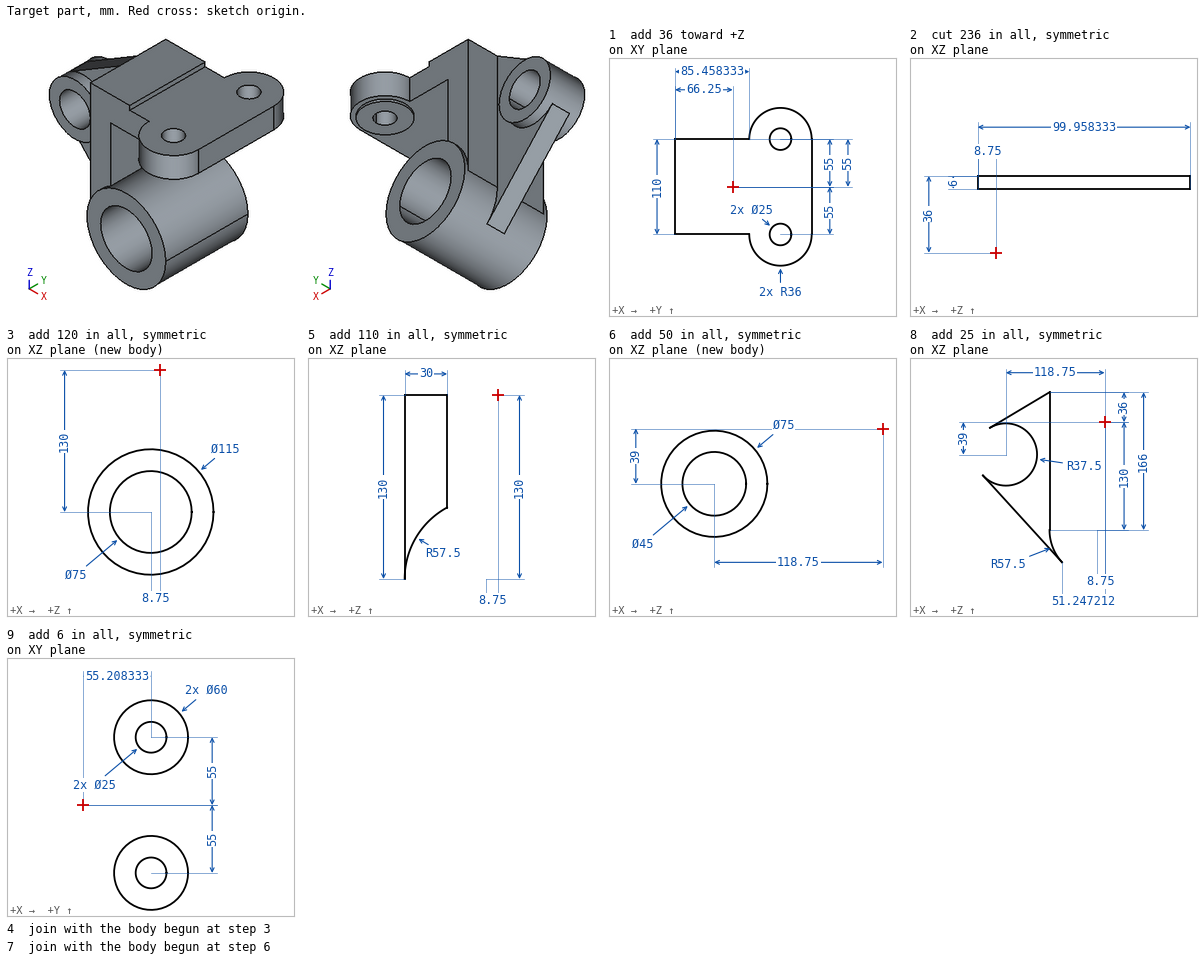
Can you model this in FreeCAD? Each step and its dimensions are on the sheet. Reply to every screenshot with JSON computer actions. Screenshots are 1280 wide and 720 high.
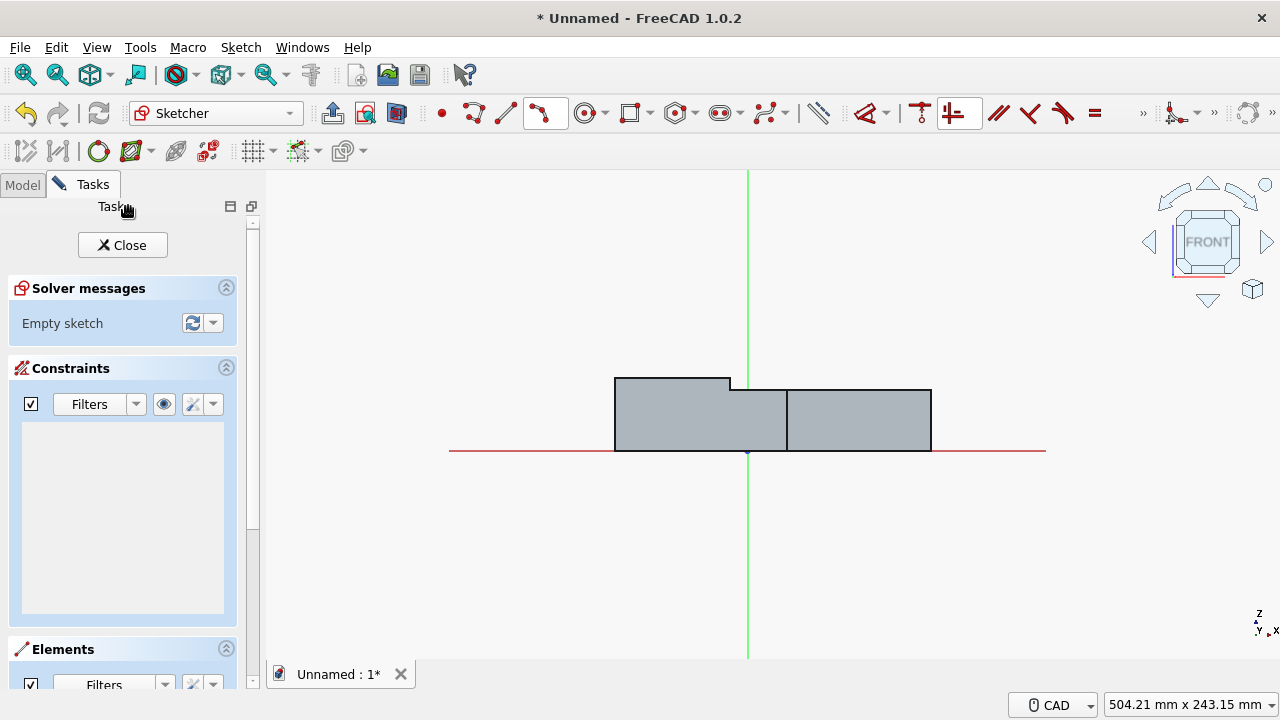
{"action": "scroll", "coordinate": [673, 198], "scroll_direction": "down", "scroll_amount": 3}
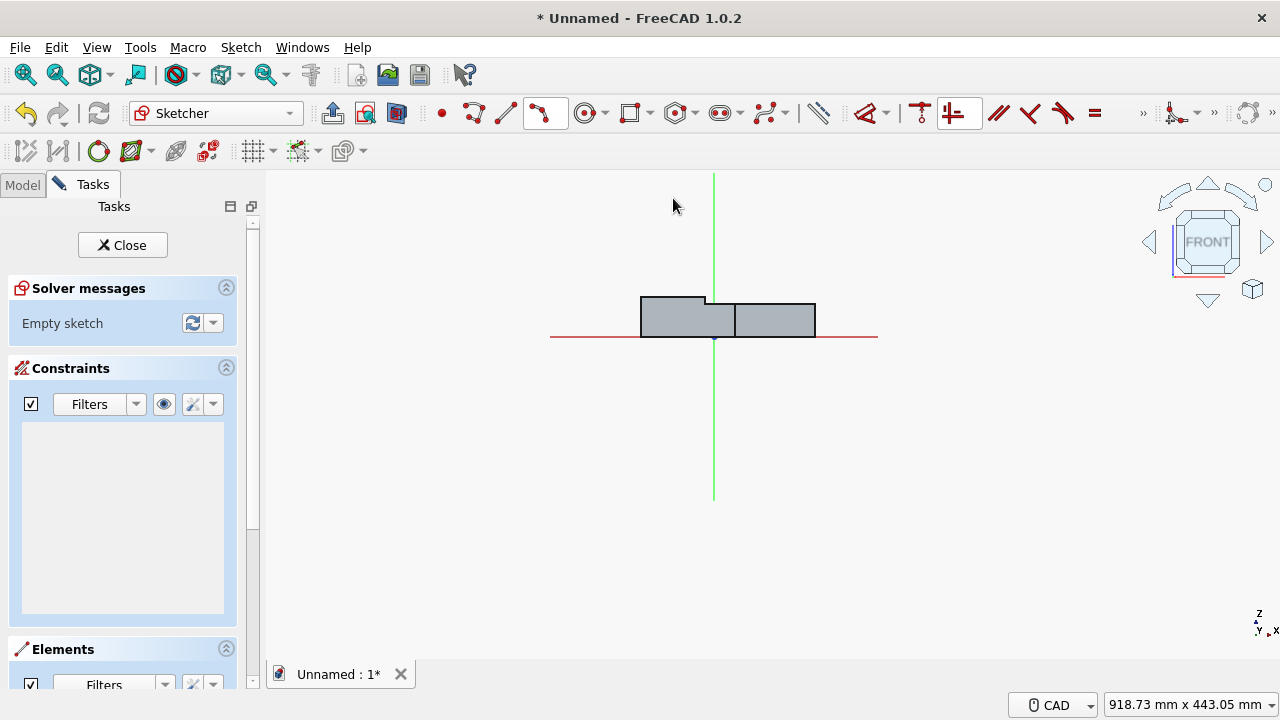
{"action": "scroll", "coordinate": [705, 492], "scroll_direction": "up", "scroll_amount": 2}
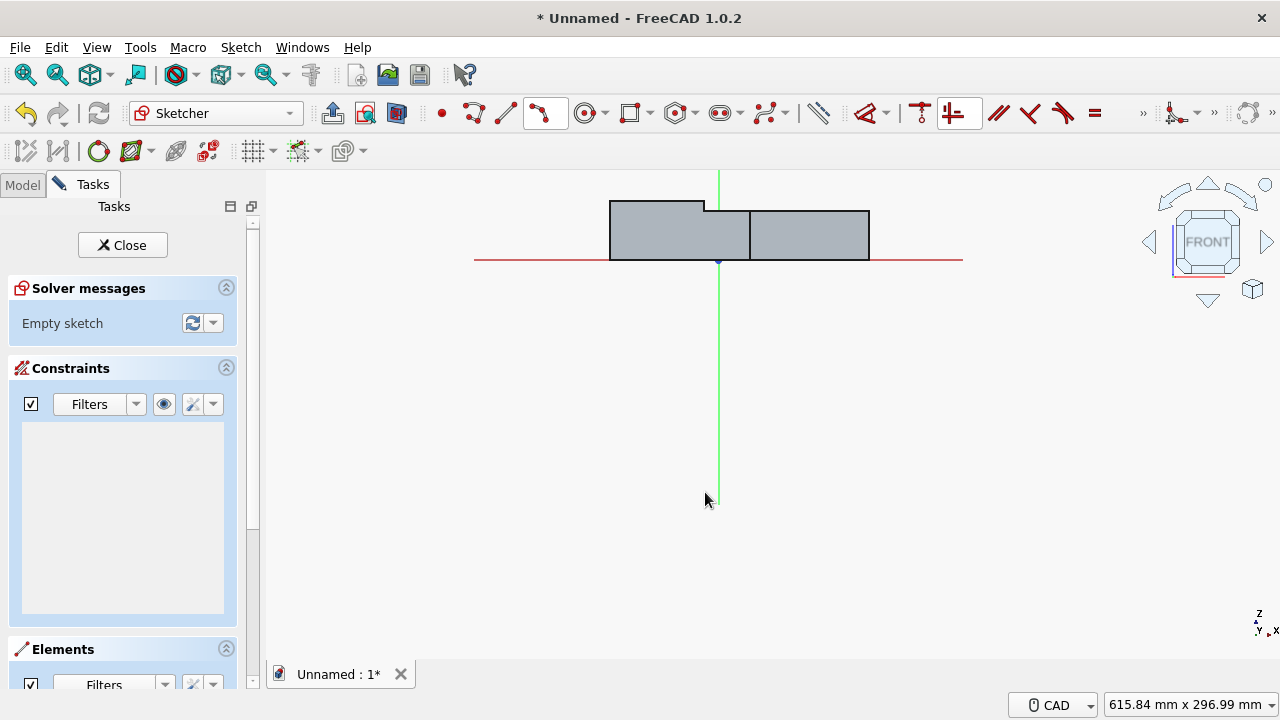
{"action": "left_click", "coordinate": [586, 114]}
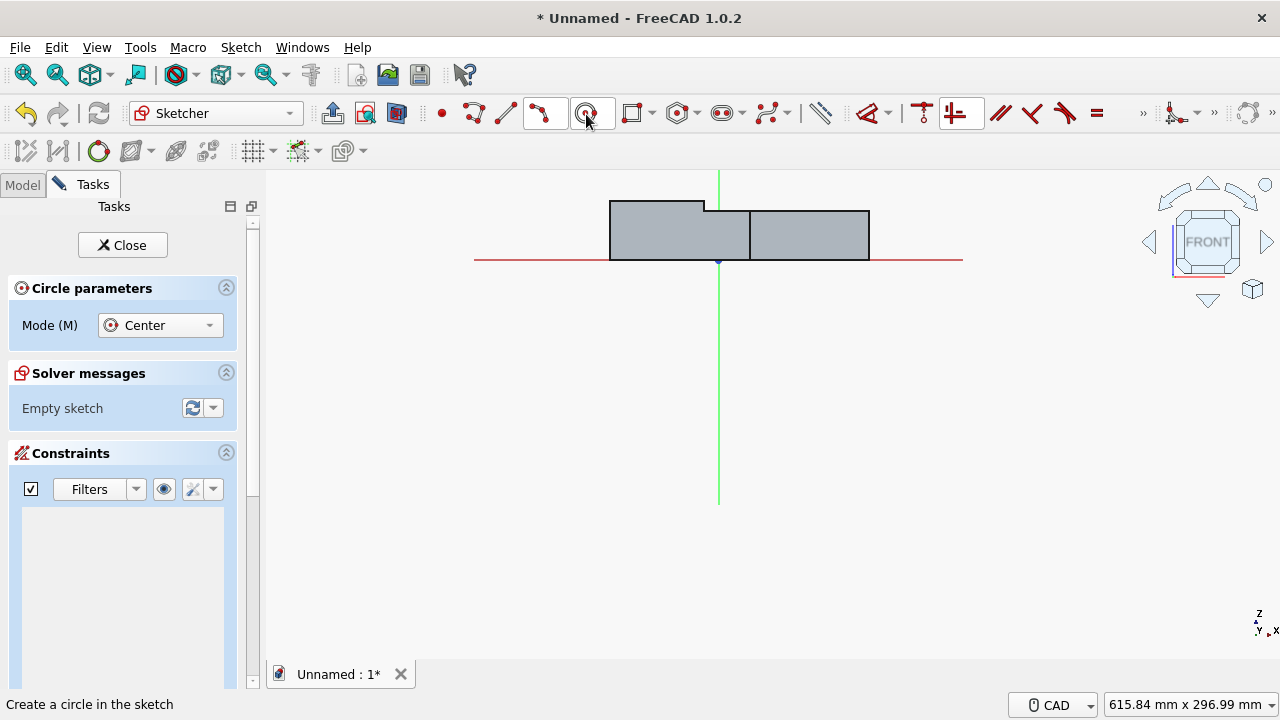
{"action": "left_click", "coordinate": [704, 474]}
{"action": "left_click", "coordinate": [771, 407]}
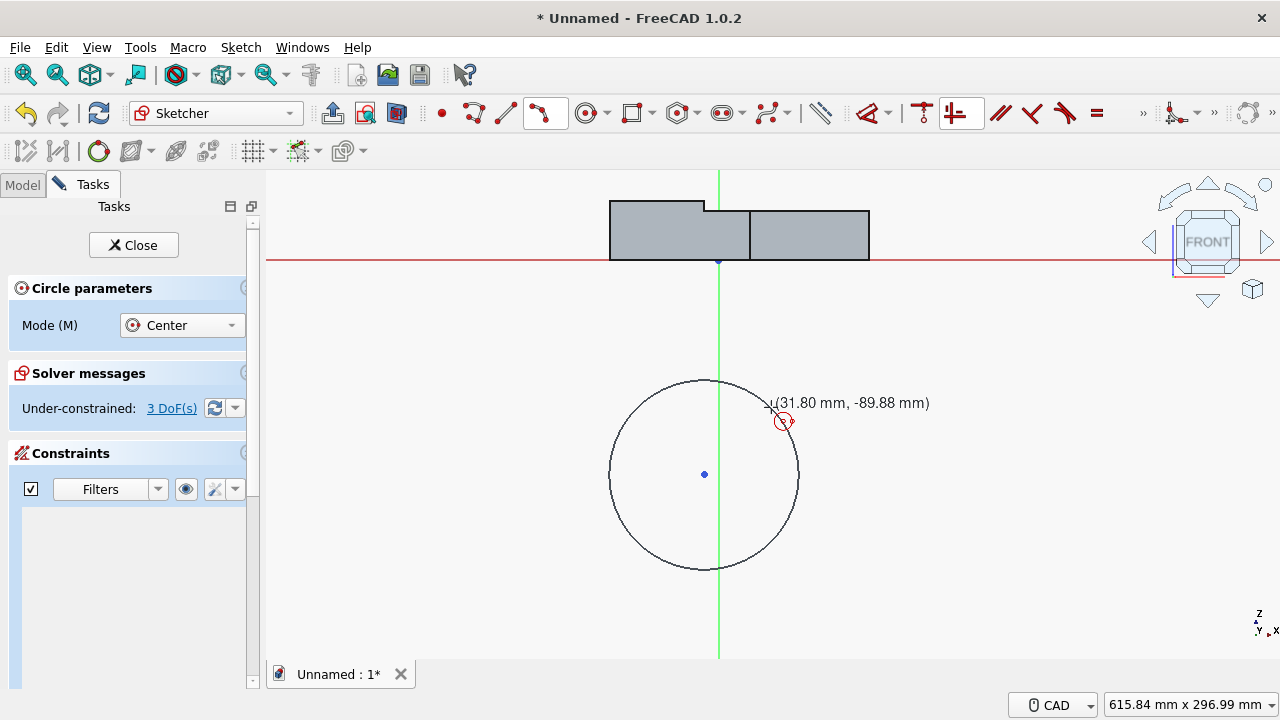
{"action": "left_click", "coordinate": [704, 475]}
{"action": "left_click", "coordinate": [748, 430]}
{"action": "key", "text": "Escape"}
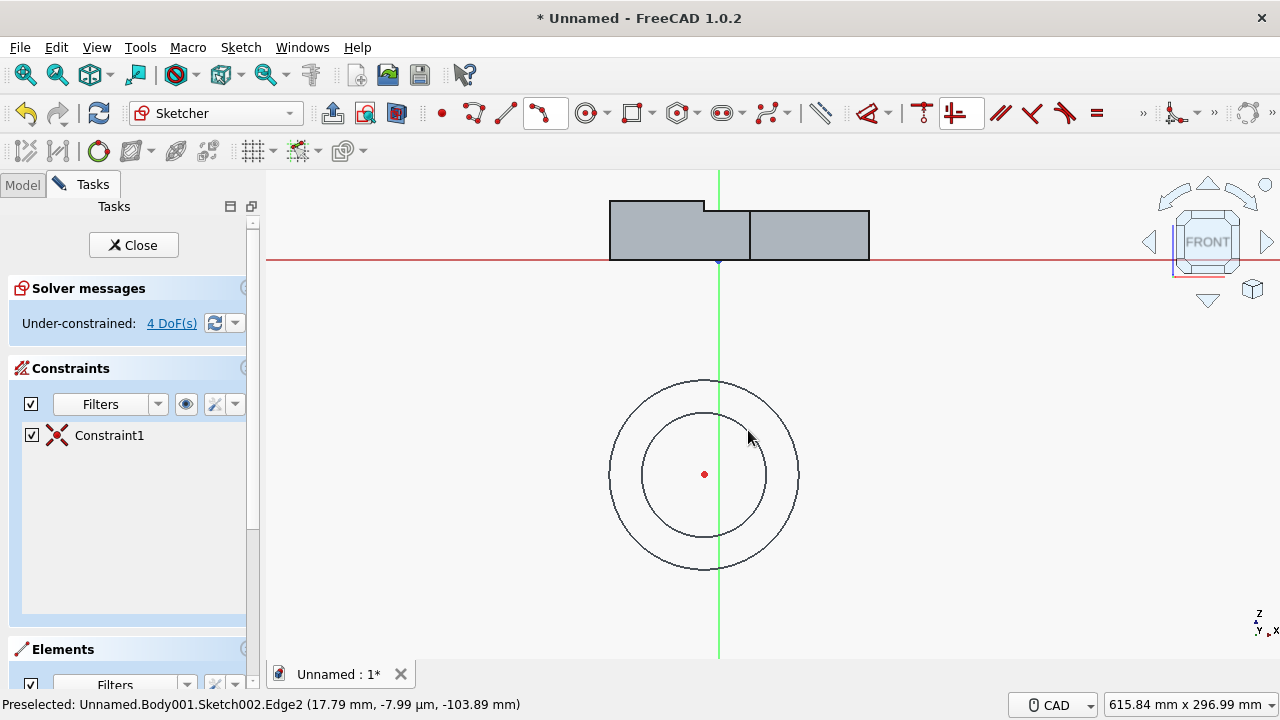
{"action": "left_click", "coordinate": [868, 114]}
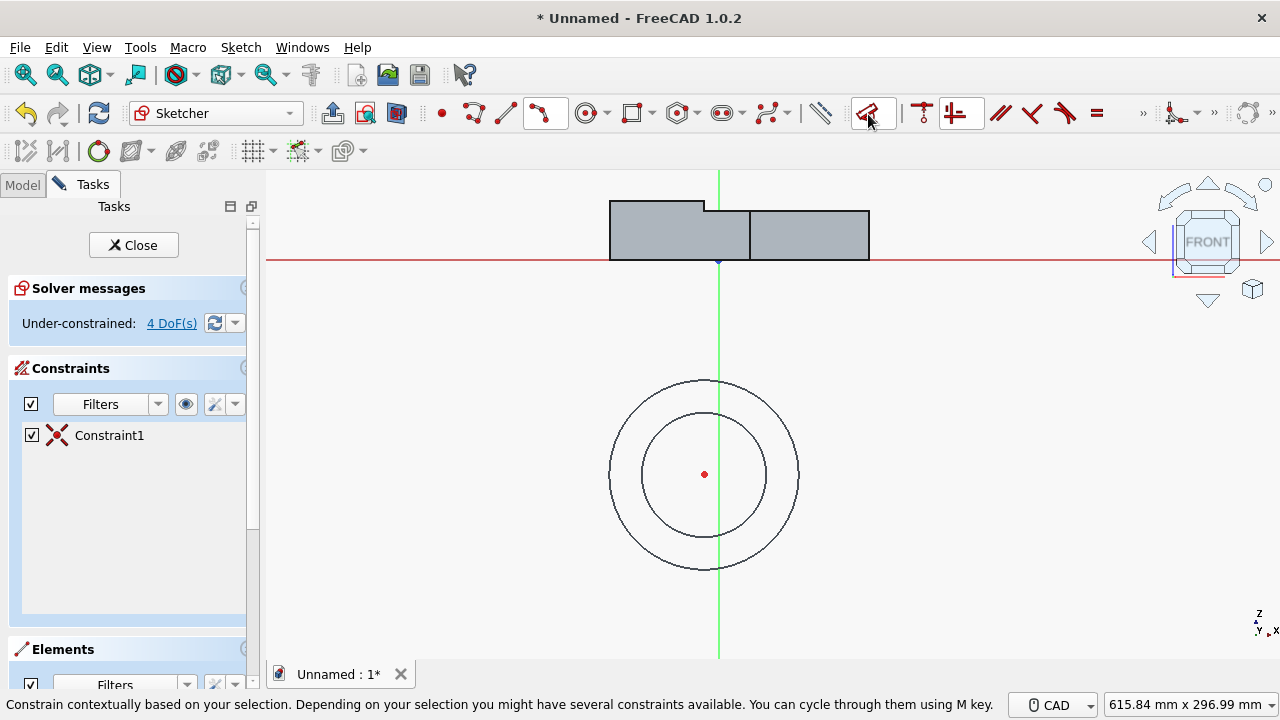
{"action": "left_click", "coordinate": [771, 408]}
{"action": "left_click", "coordinate": [794, 385]}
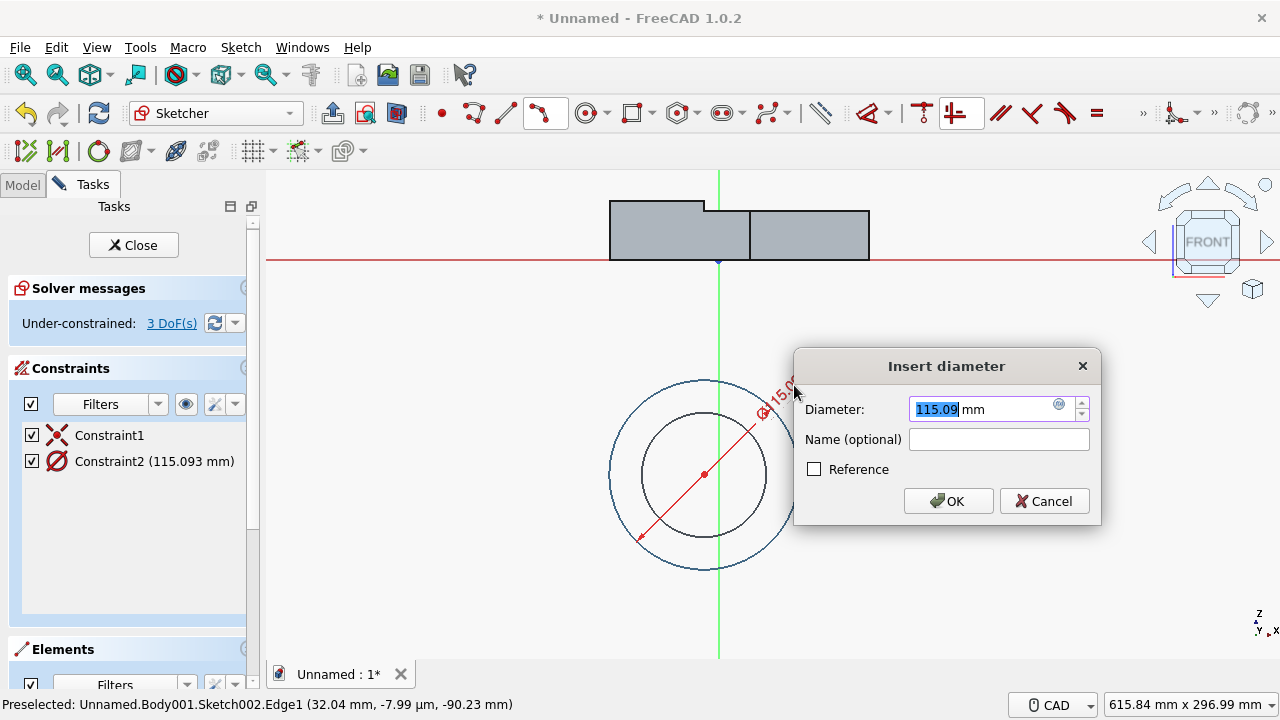
{"action": "type", "text": "115"}
{"action": "key", "text": "Return"}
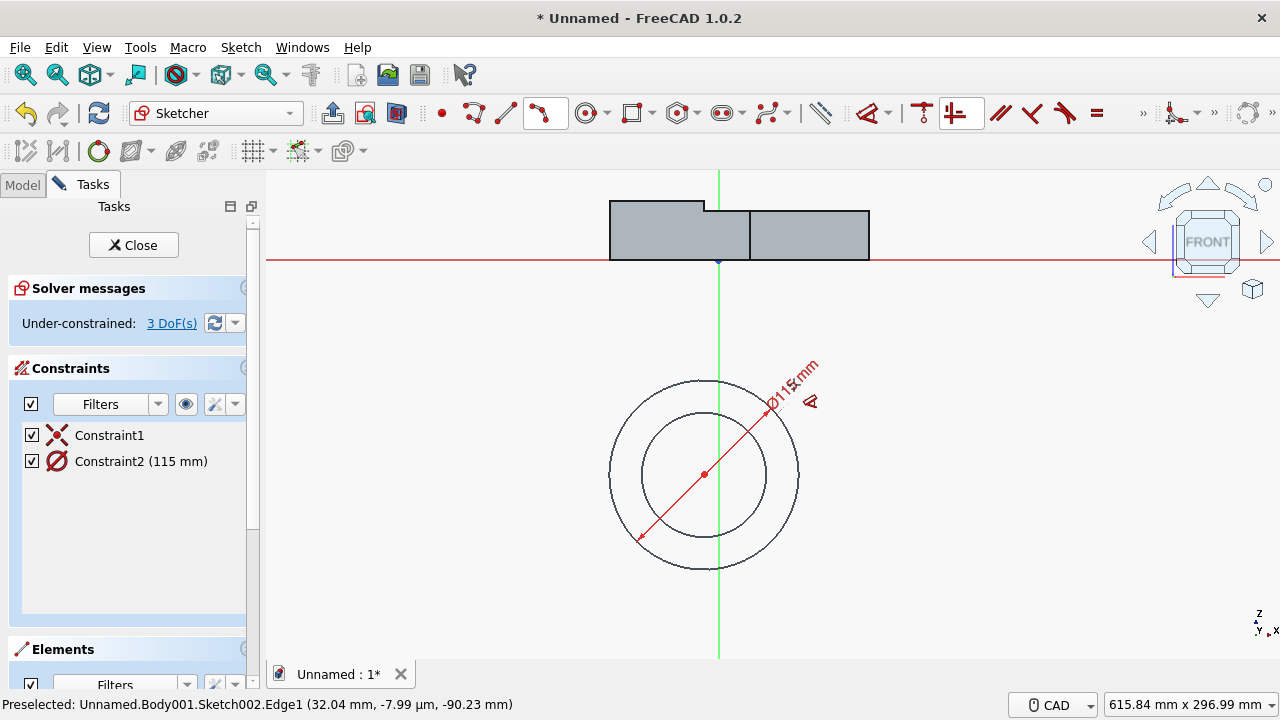
{"action": "left_click", "coordinate": [748, 431]}
{"action": "left_click", "coordinate": [816, 442]}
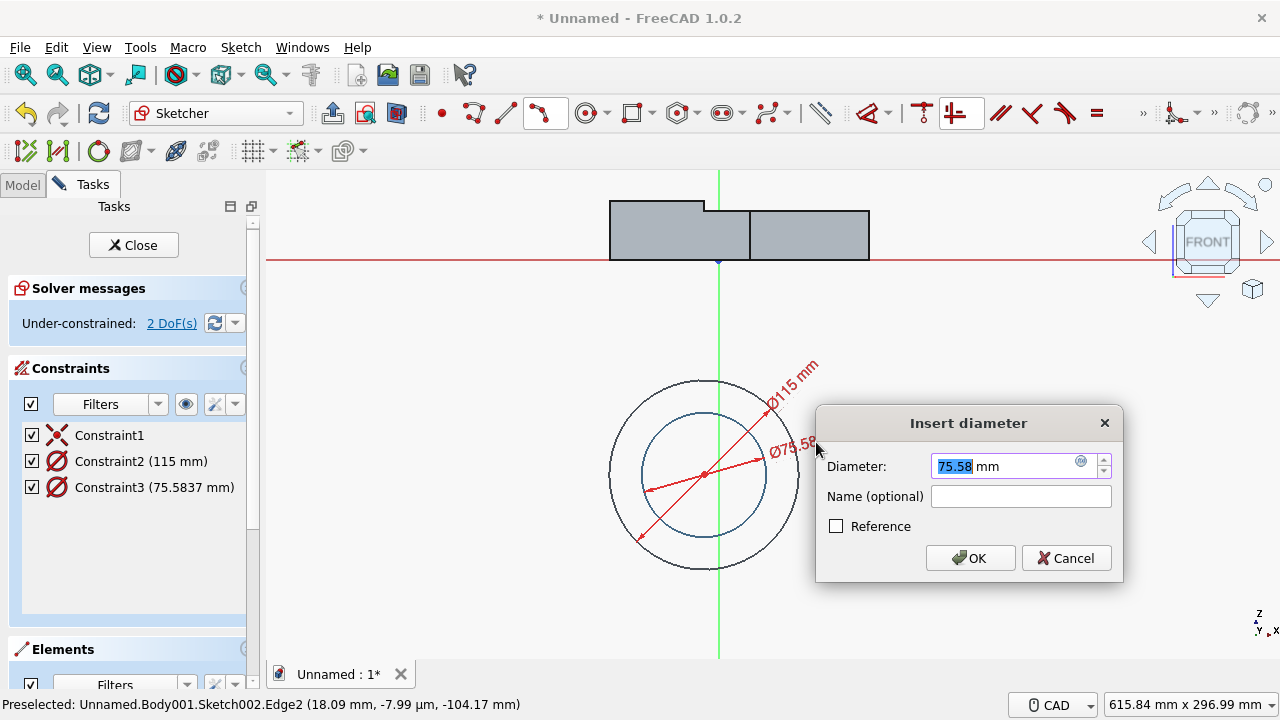
{"action": "type", "text": "75"}
{"action": "key", "text": "Return"}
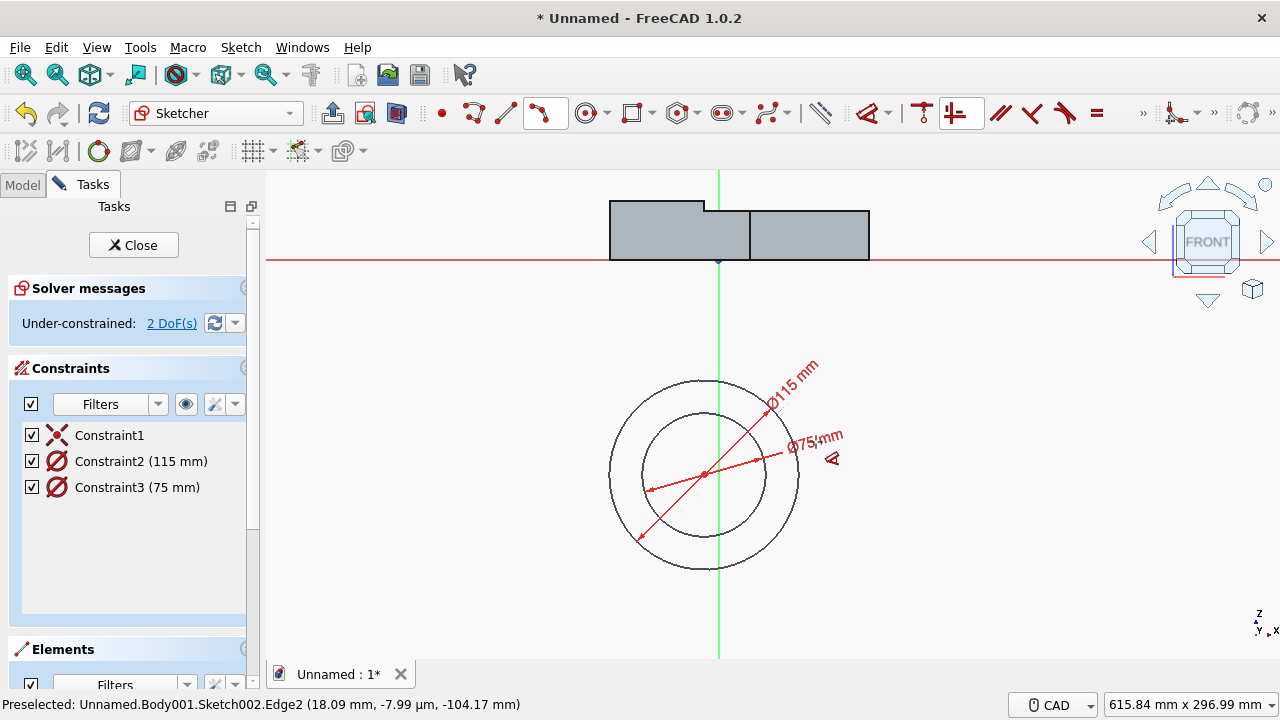
{"action": "left_click", "coordinate": [704, 475]}
{"action": "left_click", "coordinate": [753, 318]}